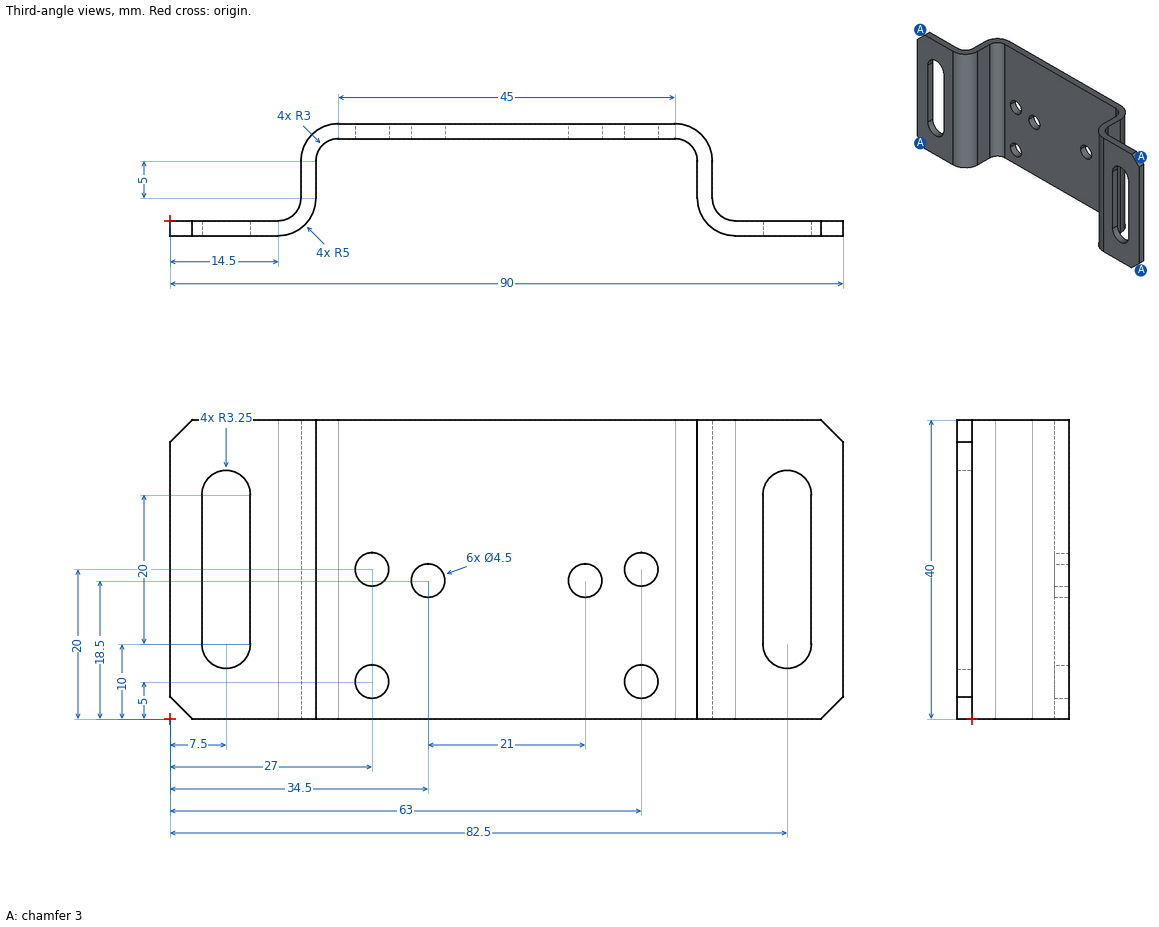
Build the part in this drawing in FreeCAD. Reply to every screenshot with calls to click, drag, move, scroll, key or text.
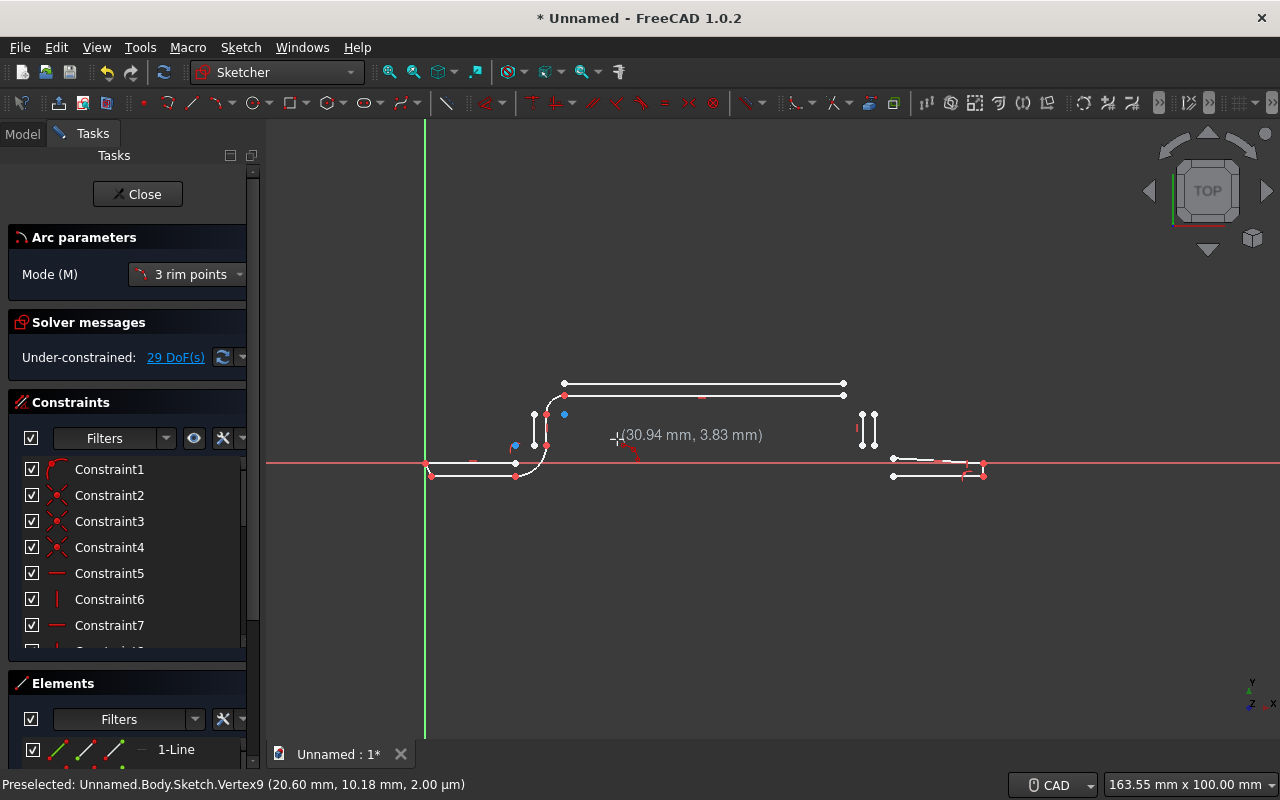
scroll(844, 395, up, 2)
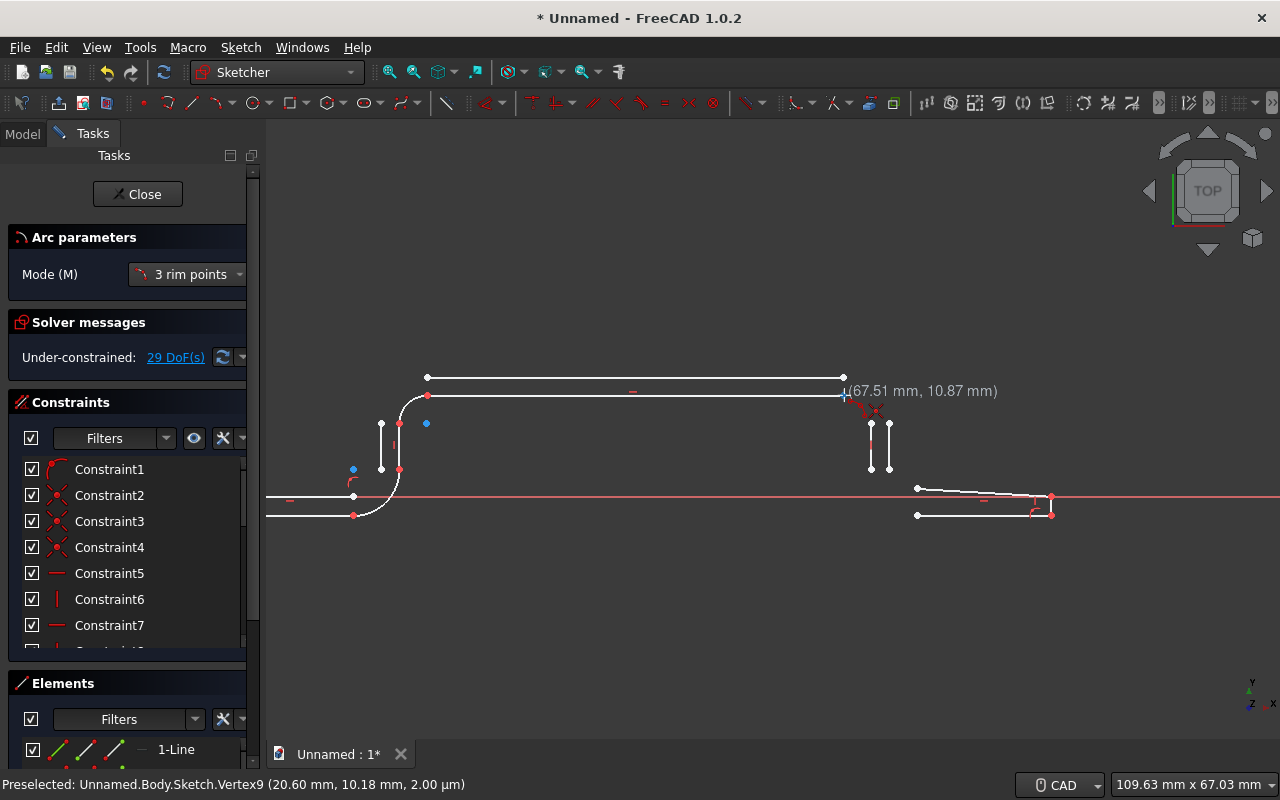
click(843, 396)
click(871, 424)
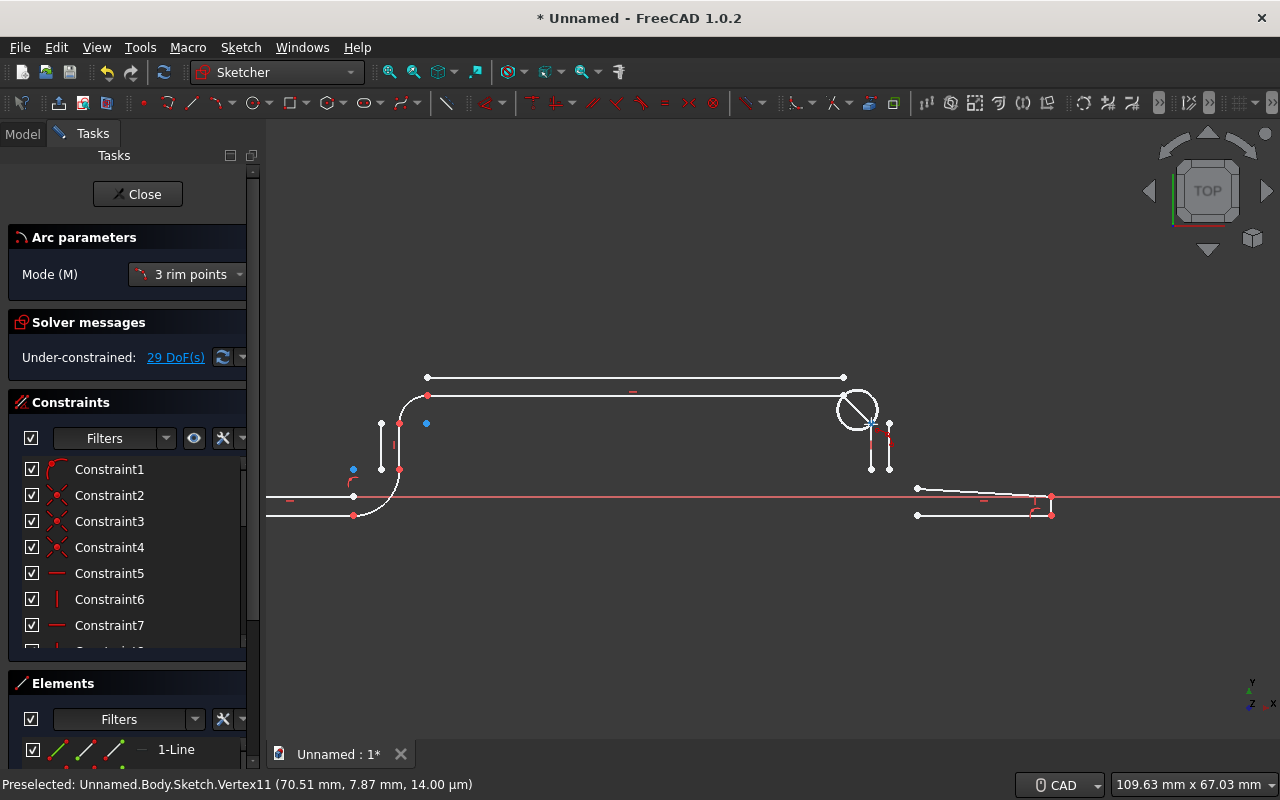
scroll(863, 403, up, 4)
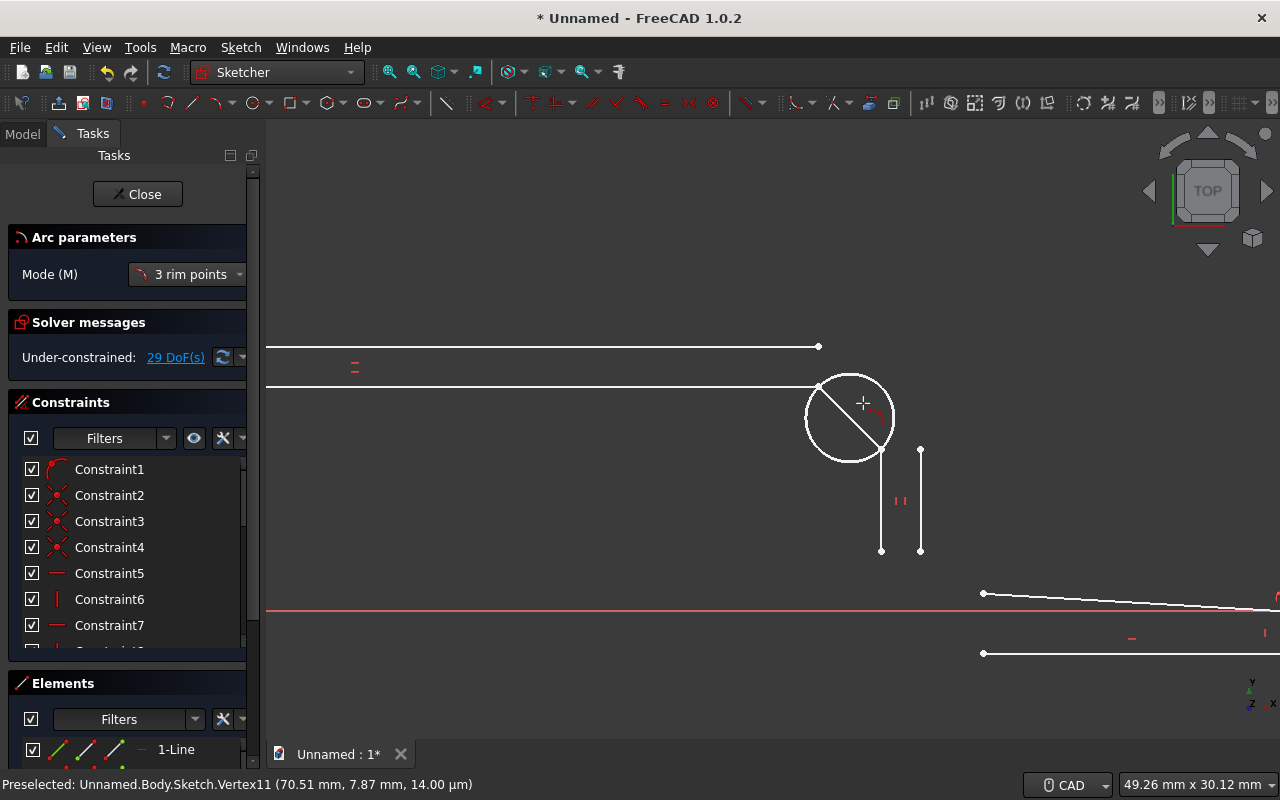
click(863, 403)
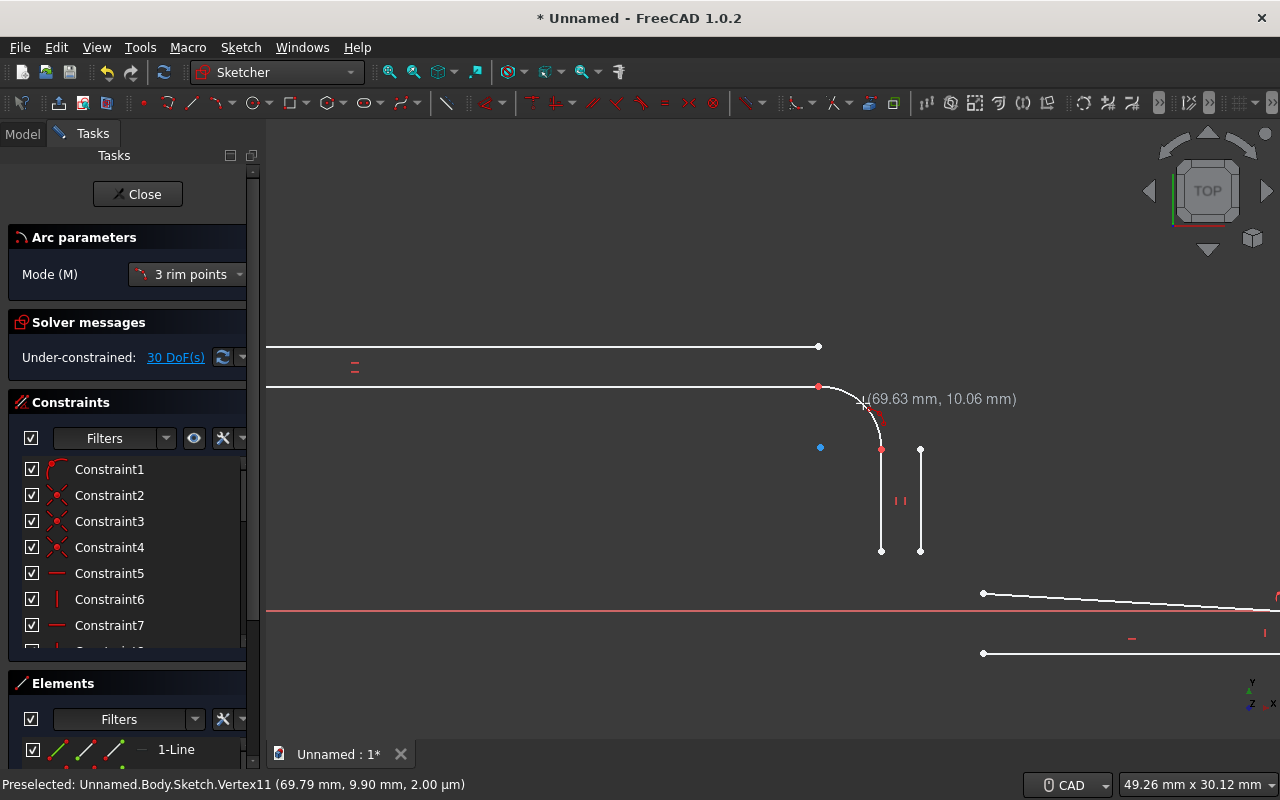
click(881, 552)
click(983, 654)
click(937, 641)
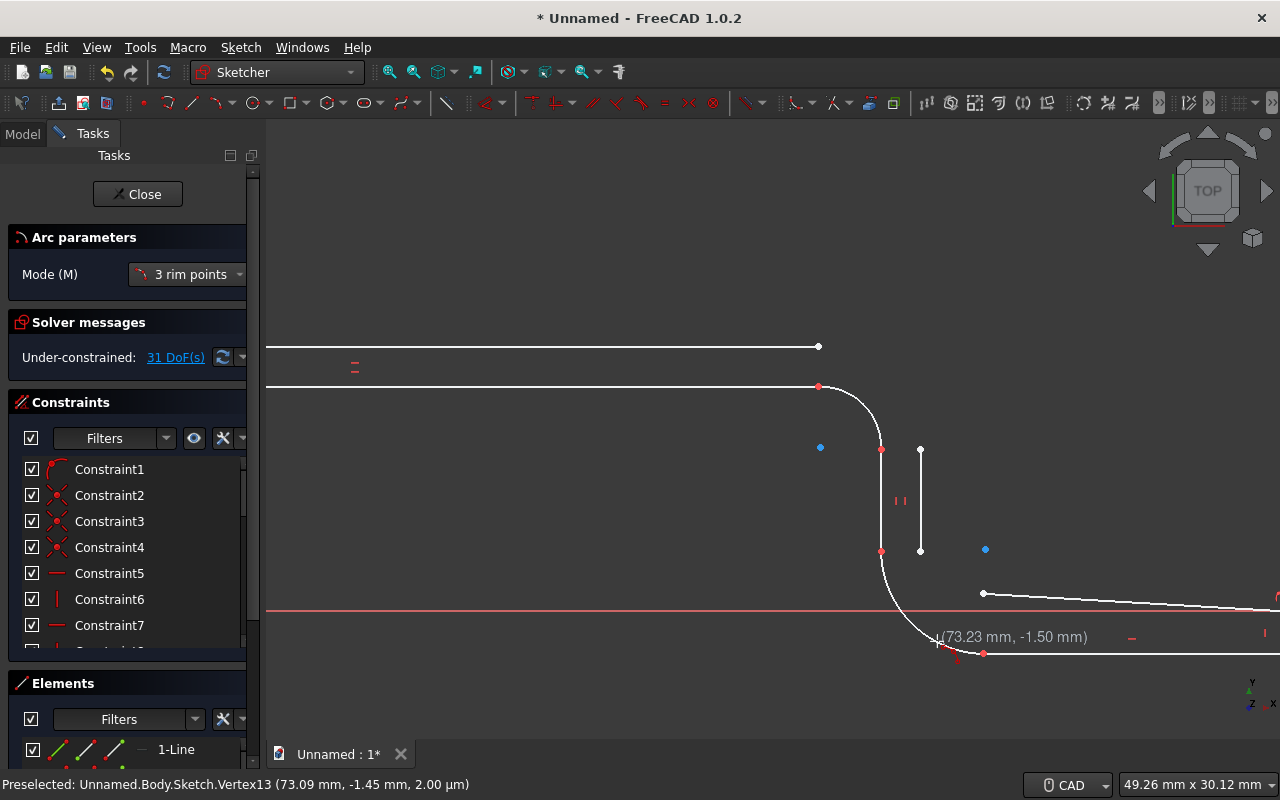
click(983, 594)
click(921, 552)
click(940, 593)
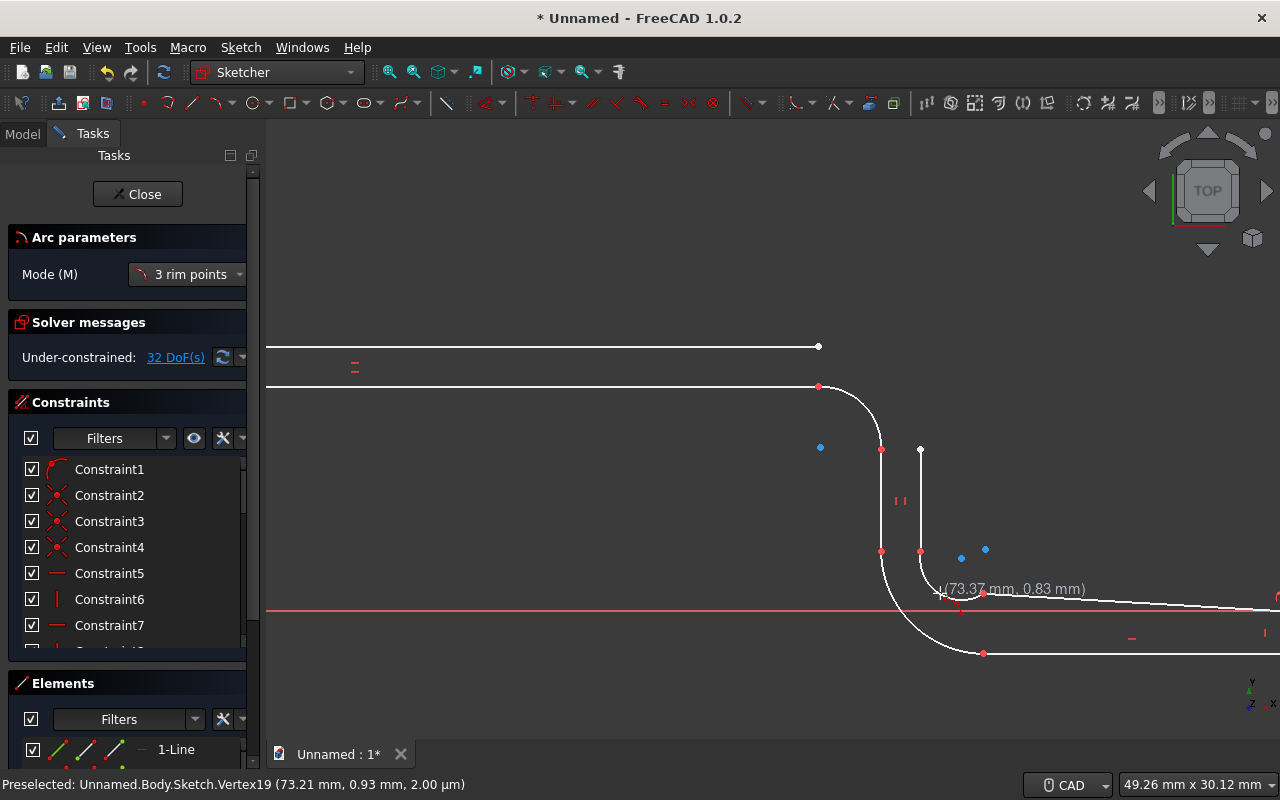
click(921, 449)
click(819, 347)
click(892, 374)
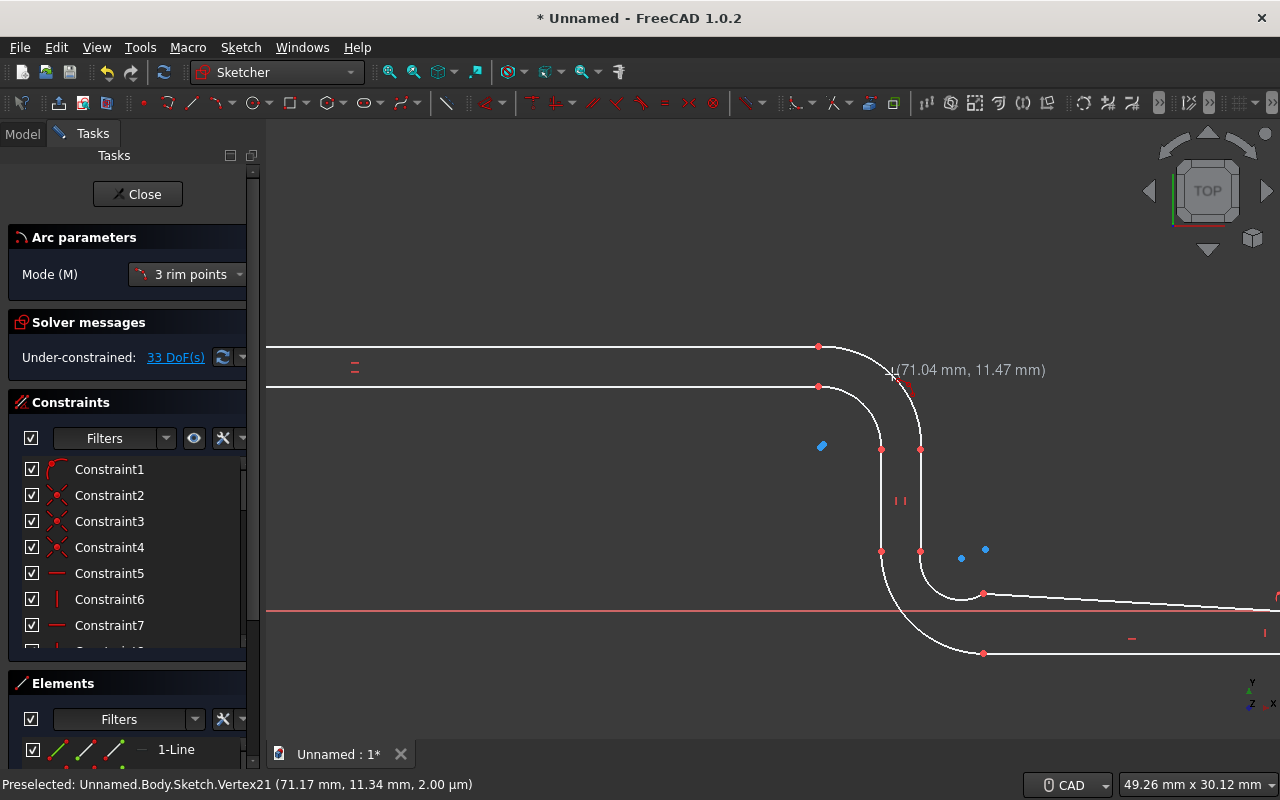
scroll(855, 399, down, 6)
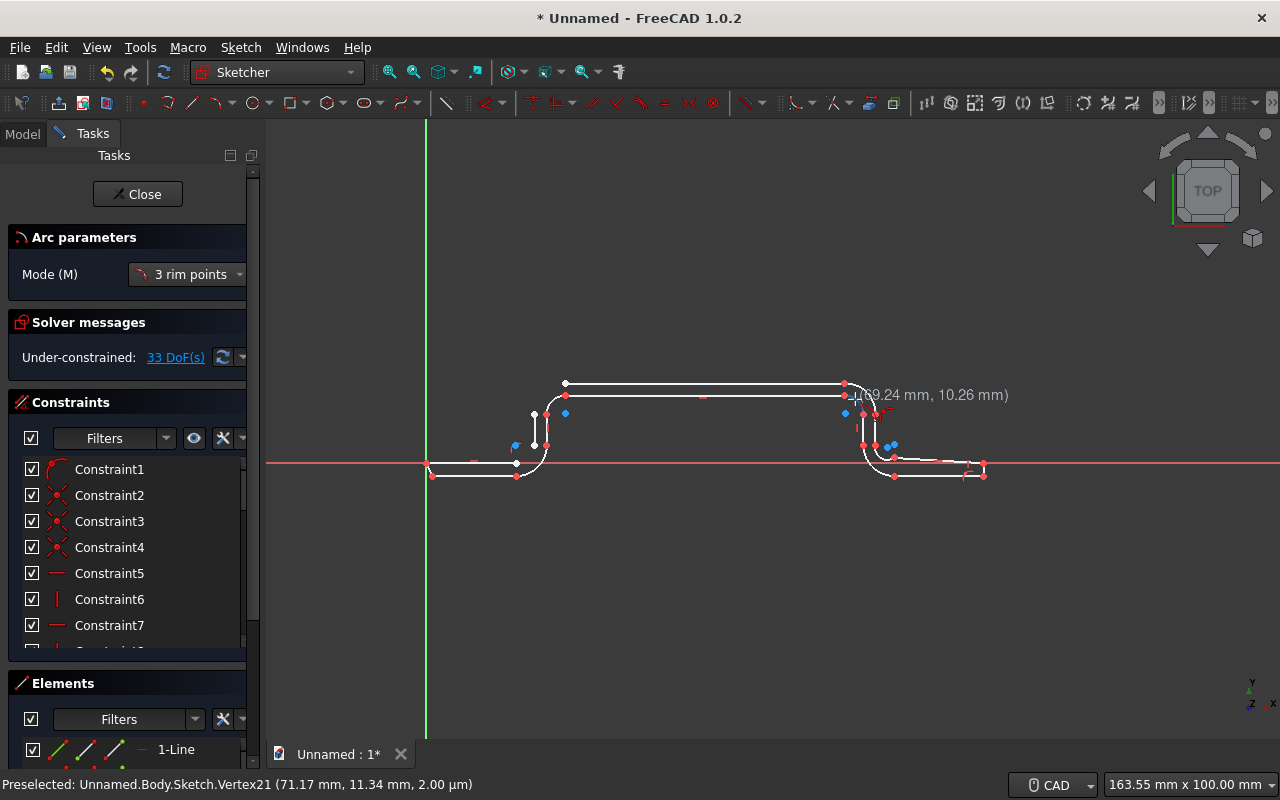
scroll(566, 383, up, 2)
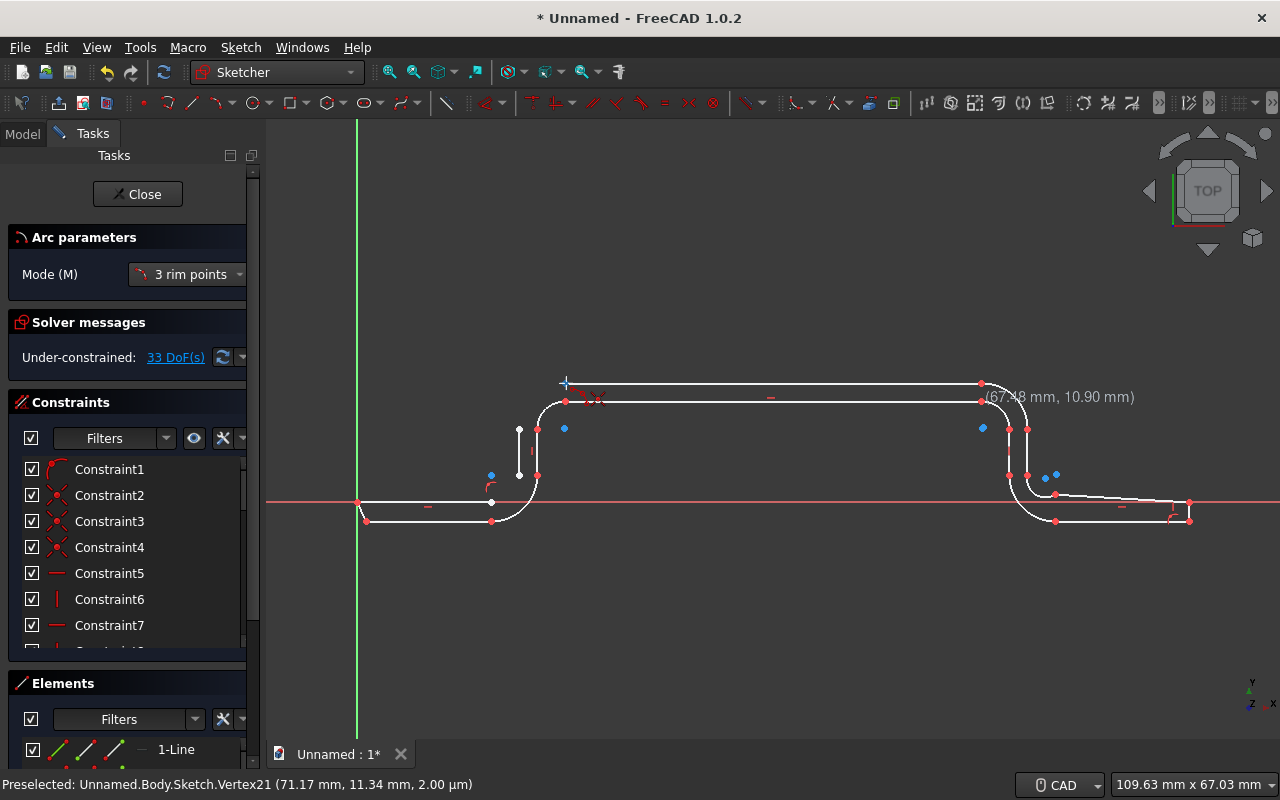
click(565, 384)
click(519, 430)
click(533, 396)